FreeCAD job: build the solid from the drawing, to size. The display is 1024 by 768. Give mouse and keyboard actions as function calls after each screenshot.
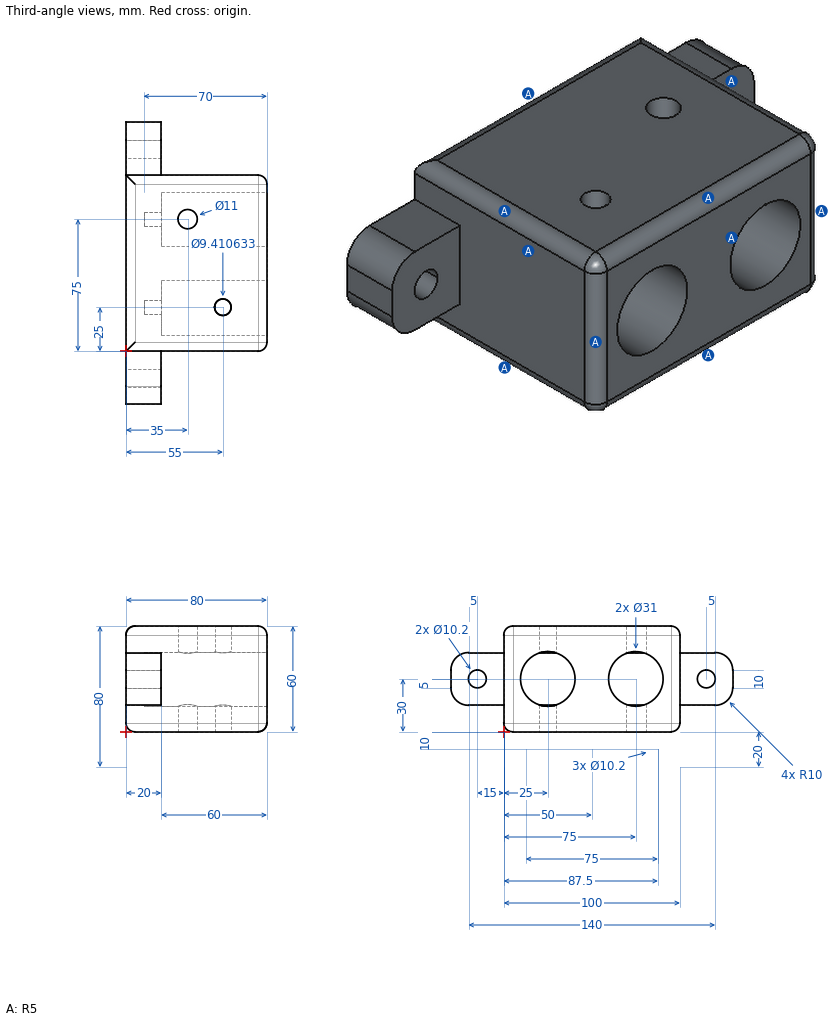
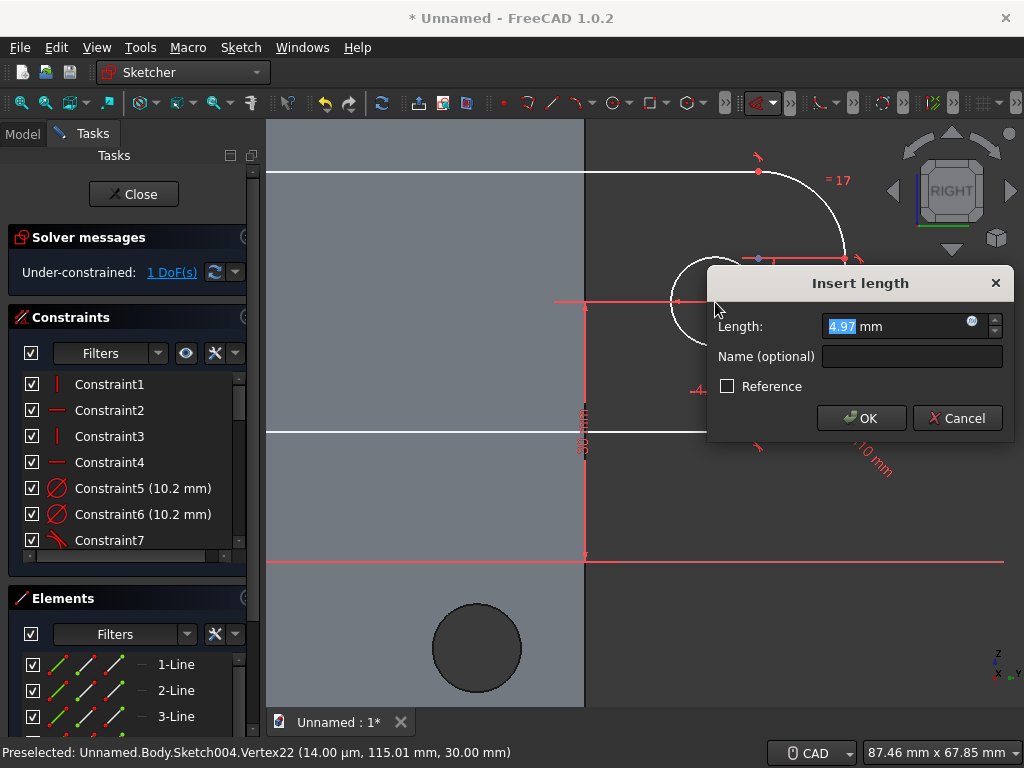
text(5)
key(Return)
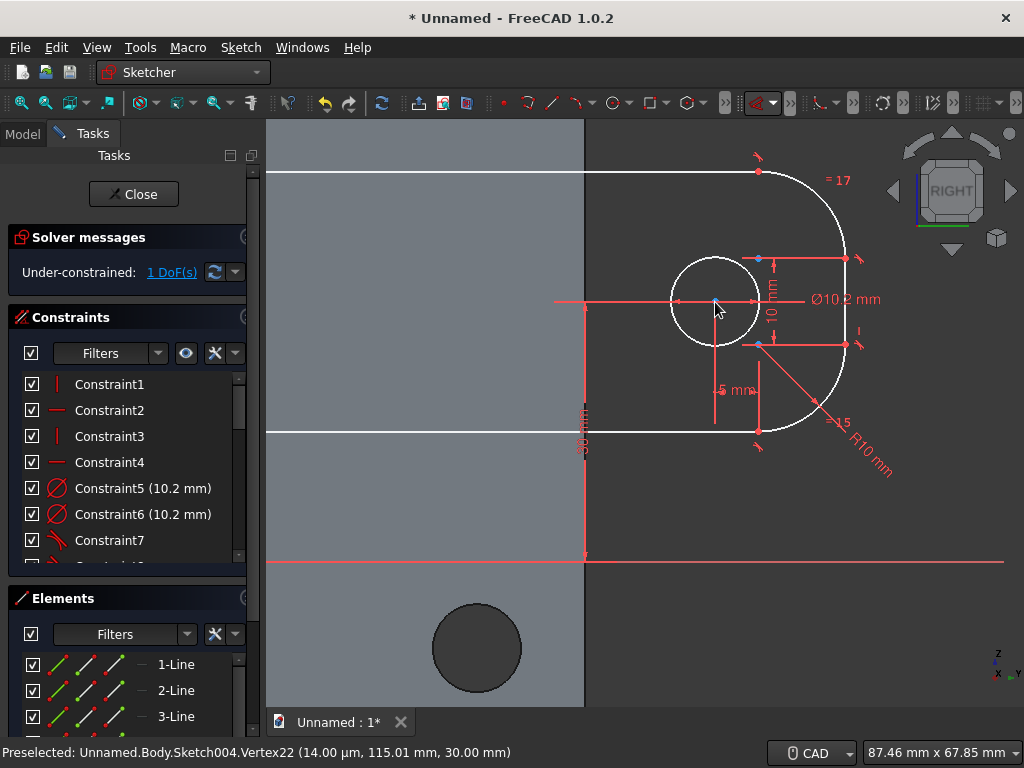
click(395, 432)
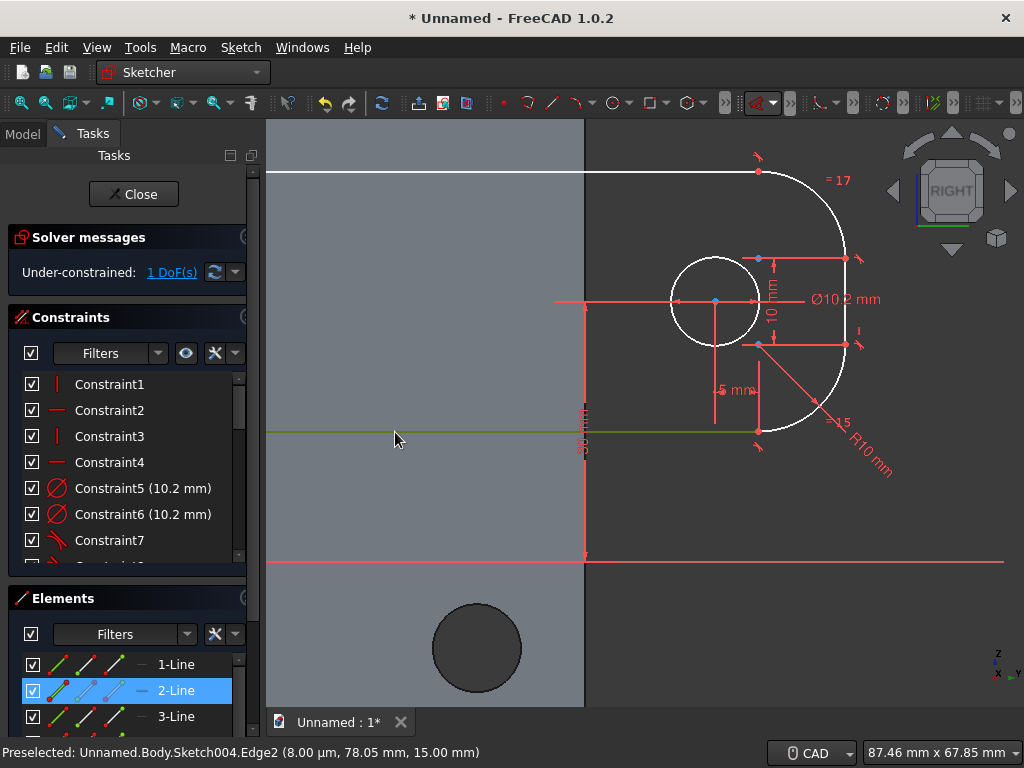
key(l)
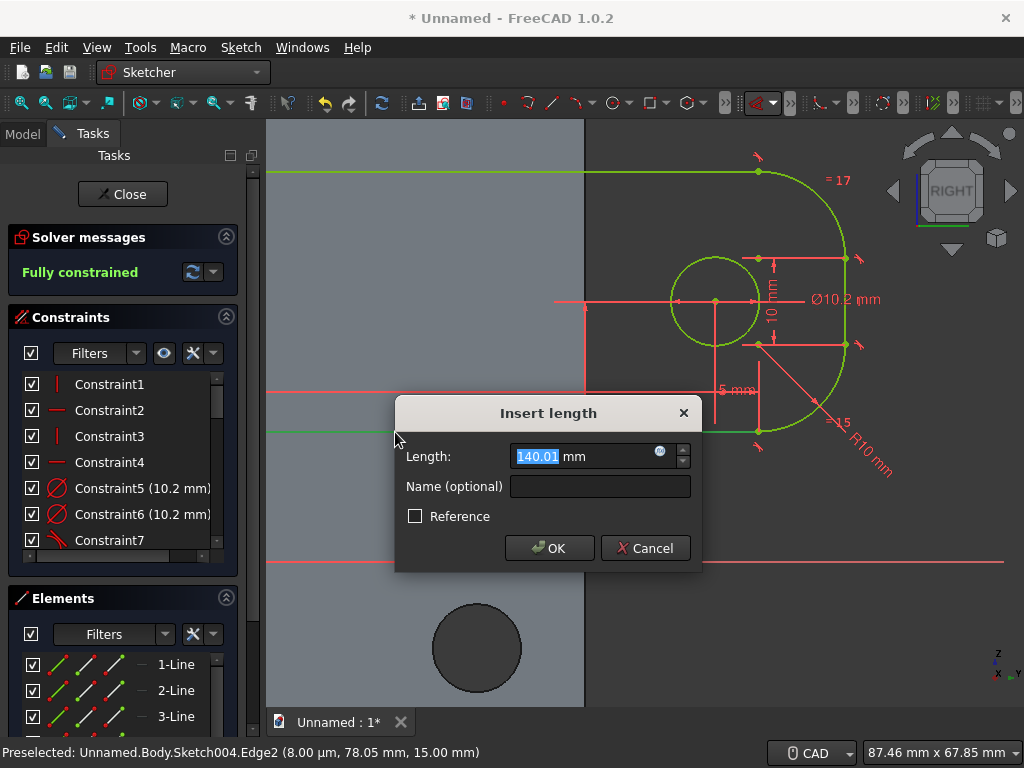
text(140)
key(Return)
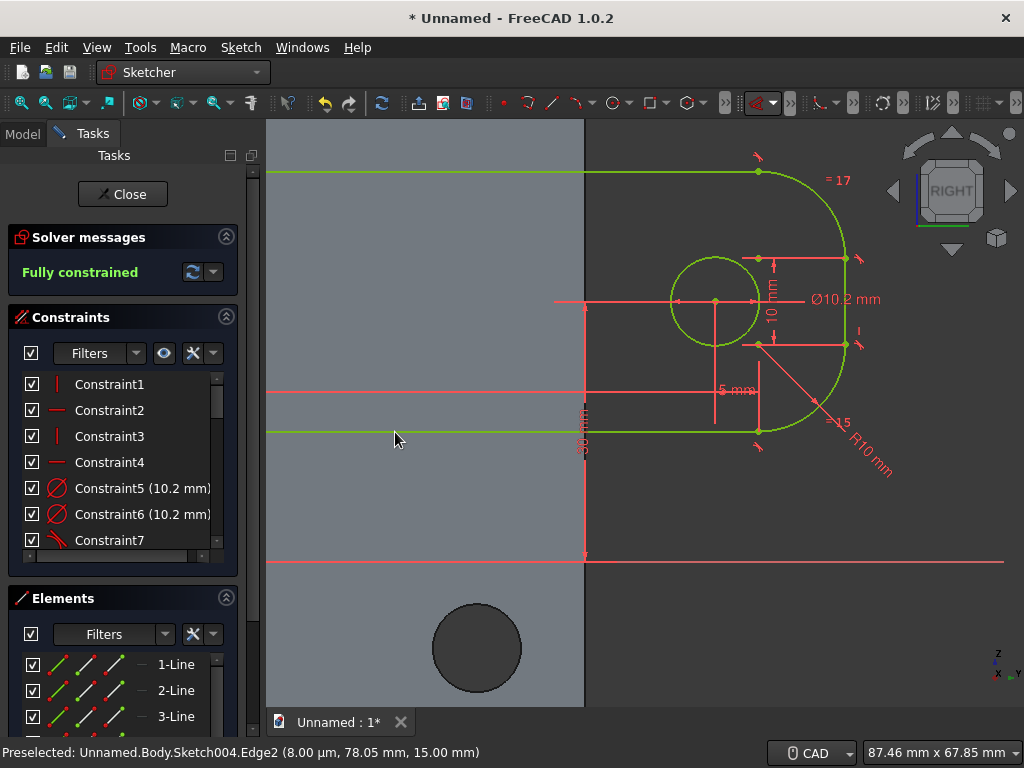
click(123, 194)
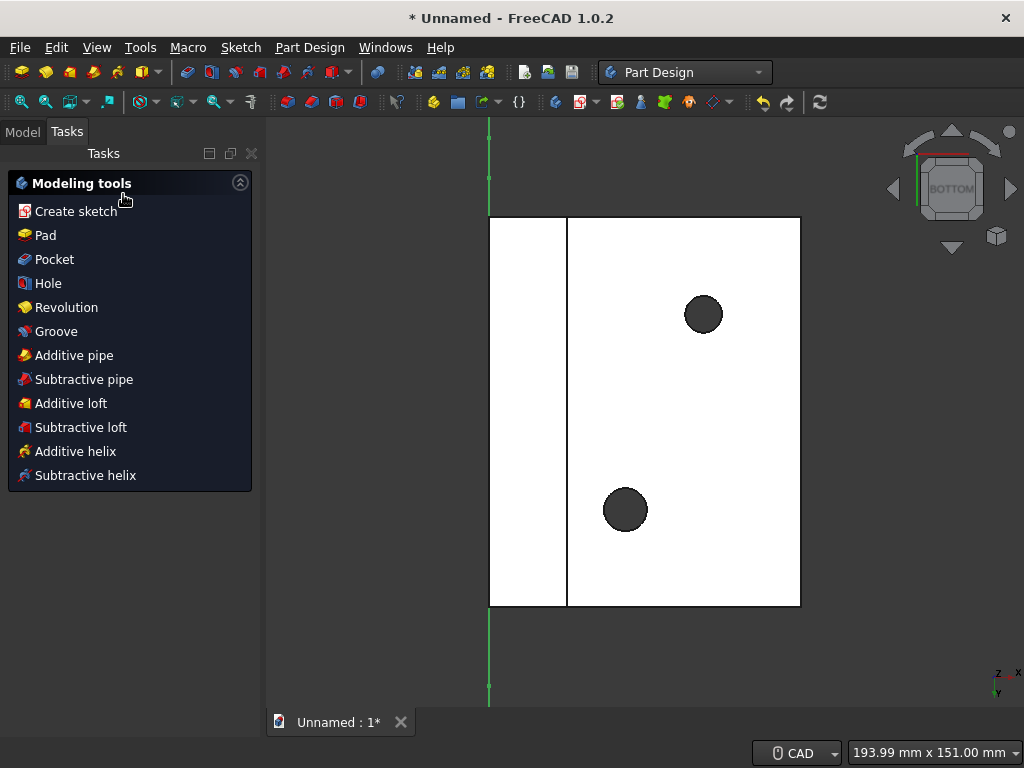
click(22, 72)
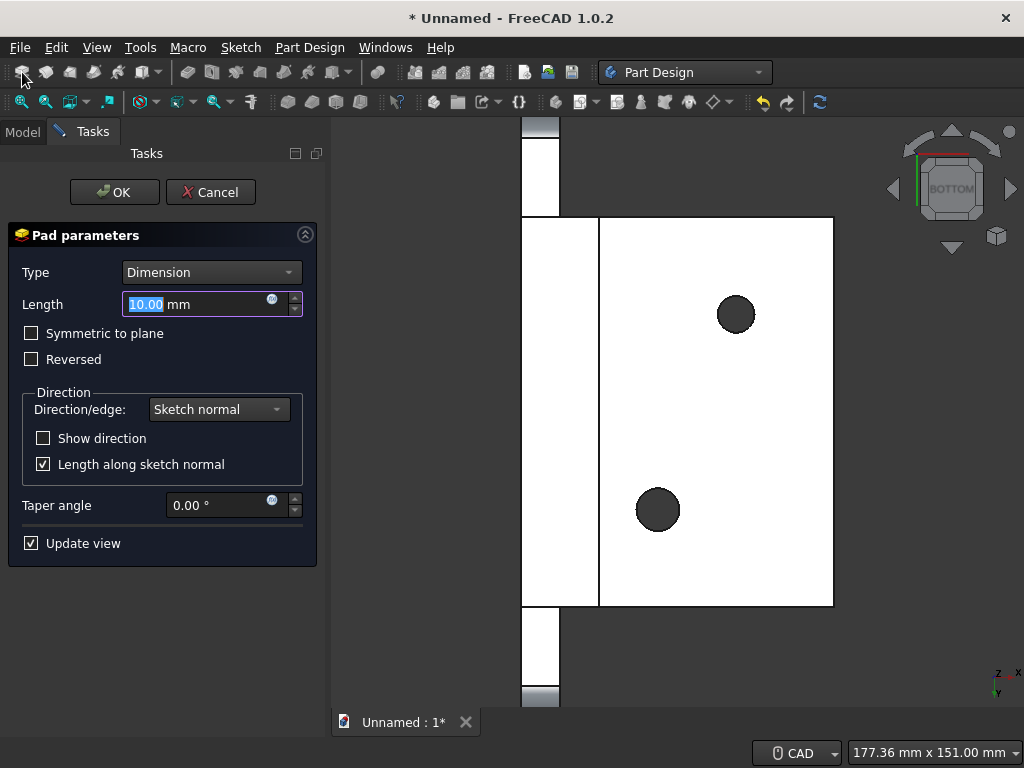
text(20)
key(Tab)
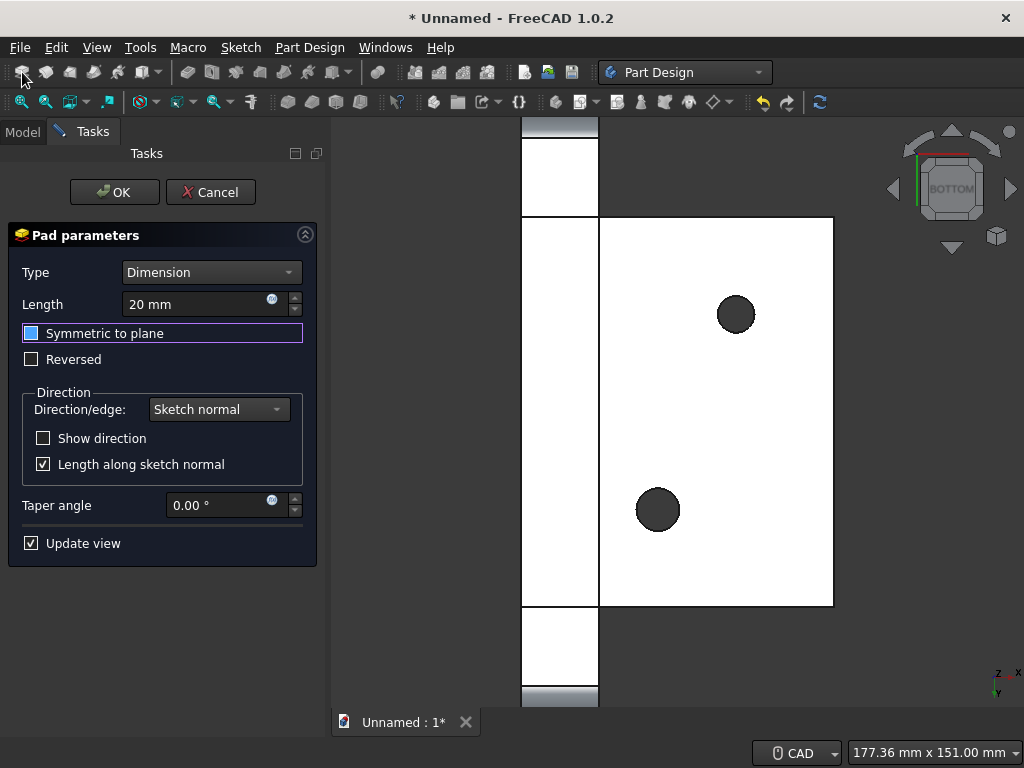
click(115, 192)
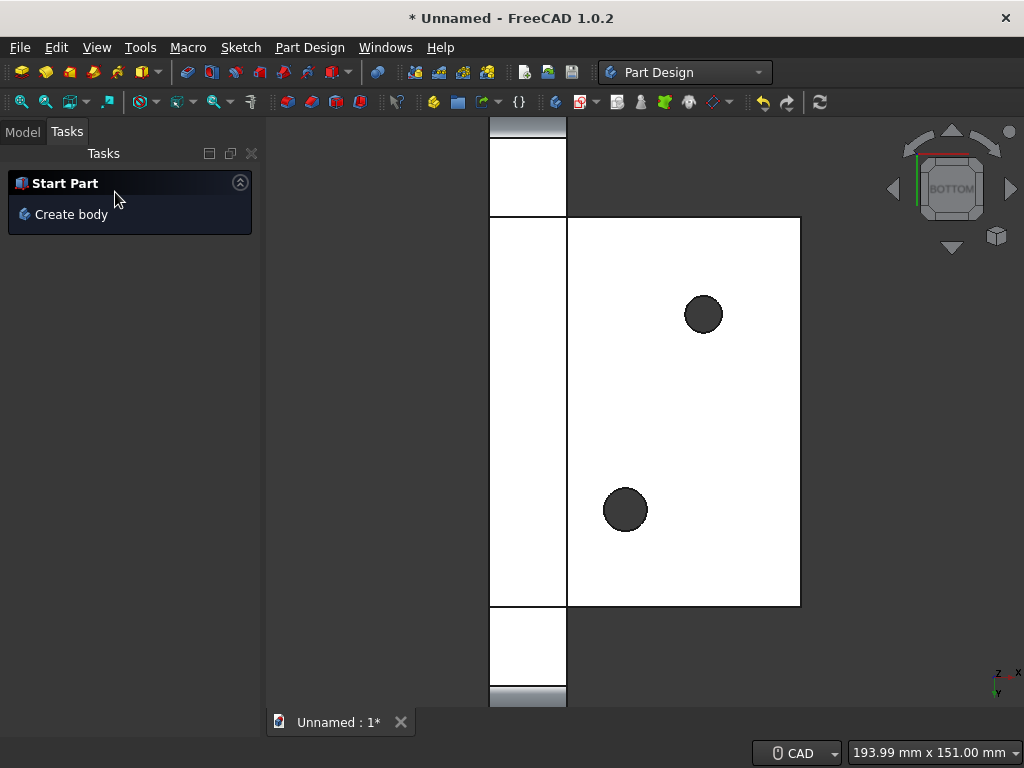
key(v)
key(f)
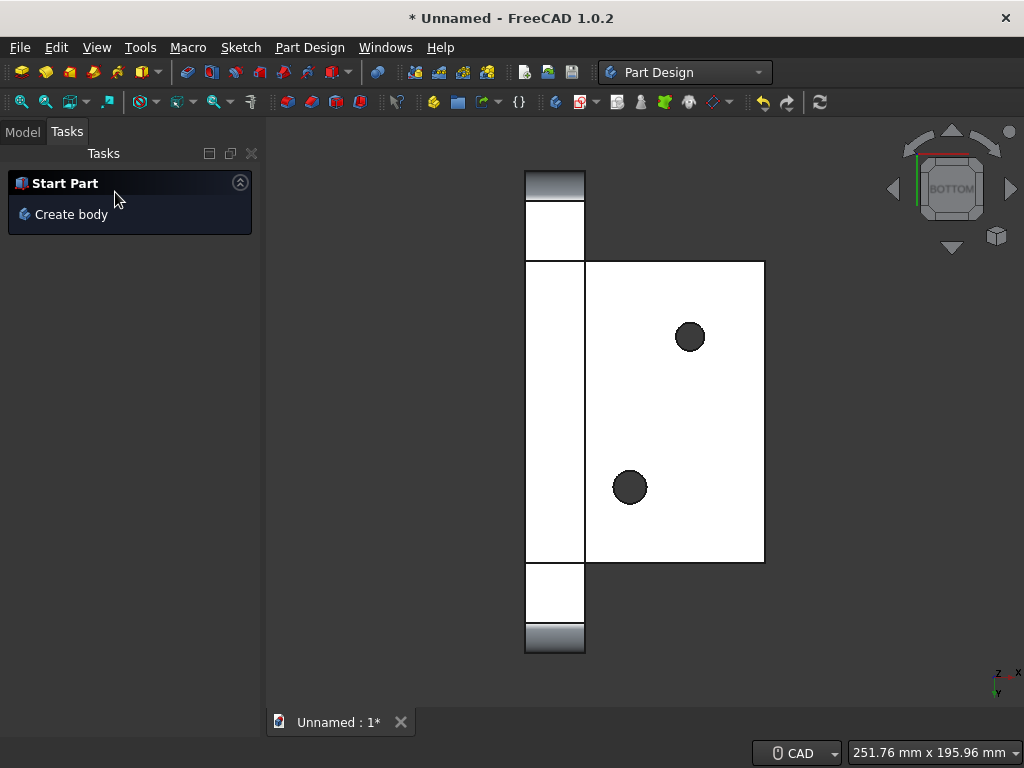
key(0)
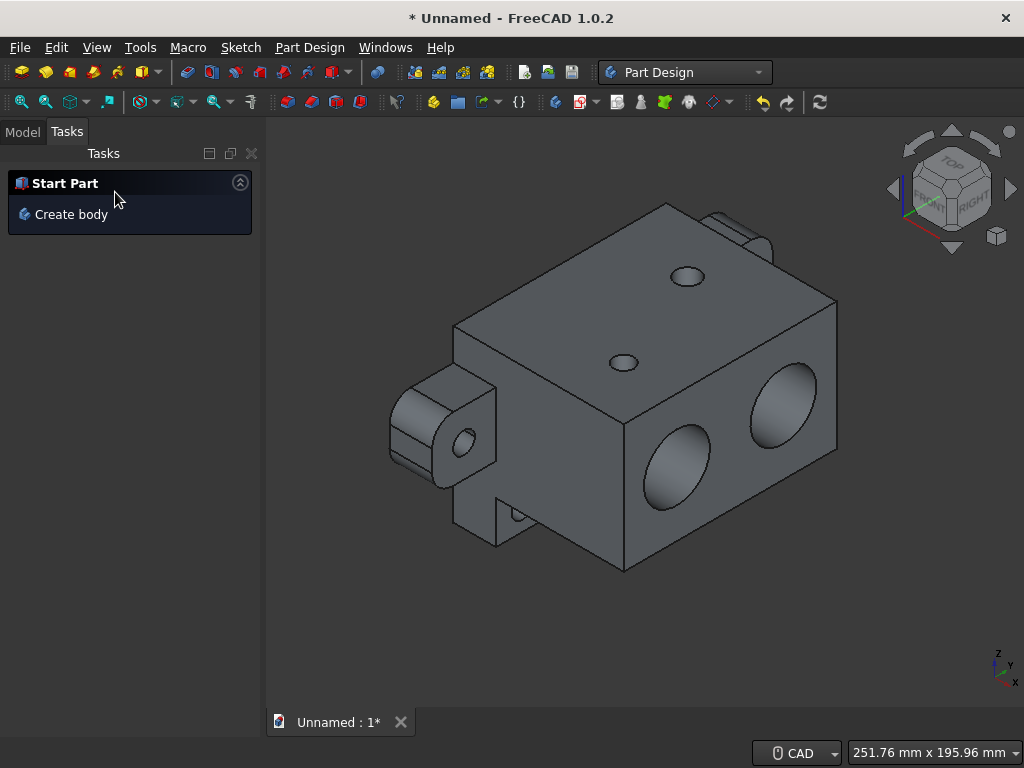
key(3)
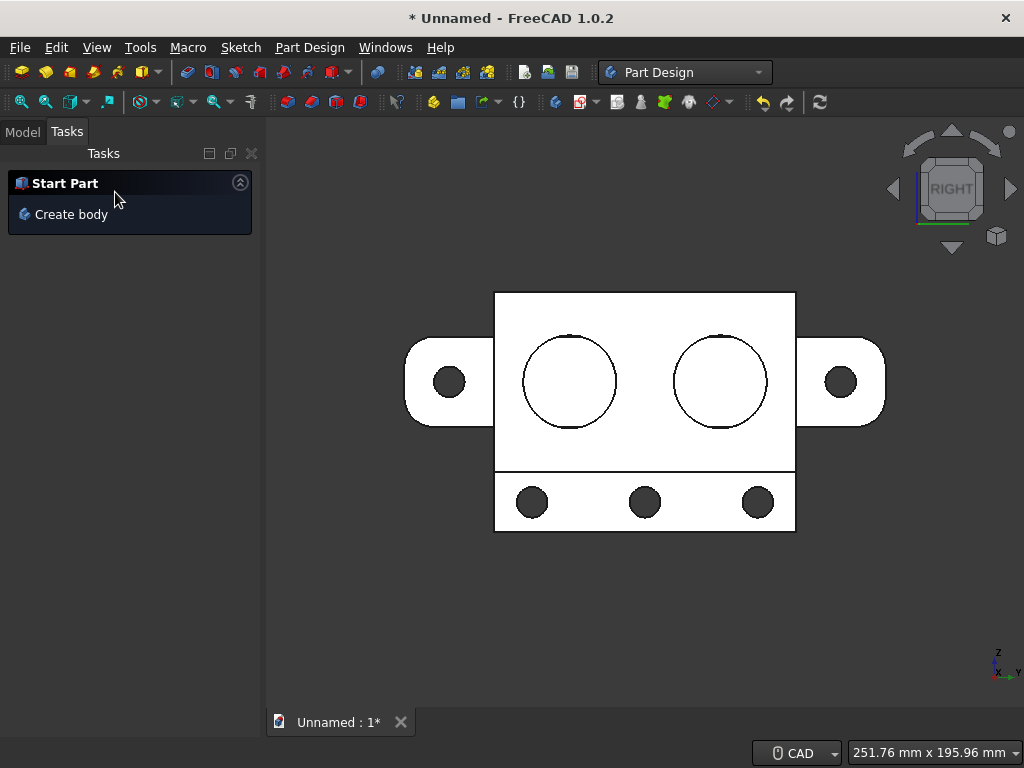
click(688, 501)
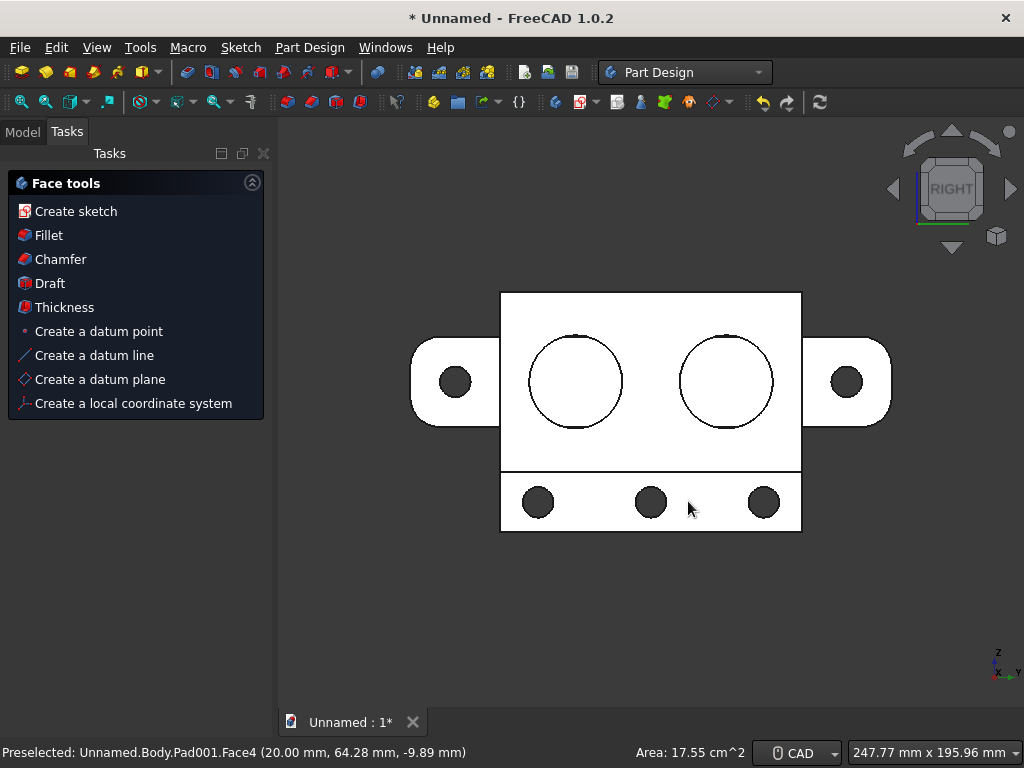
click(580, 102)